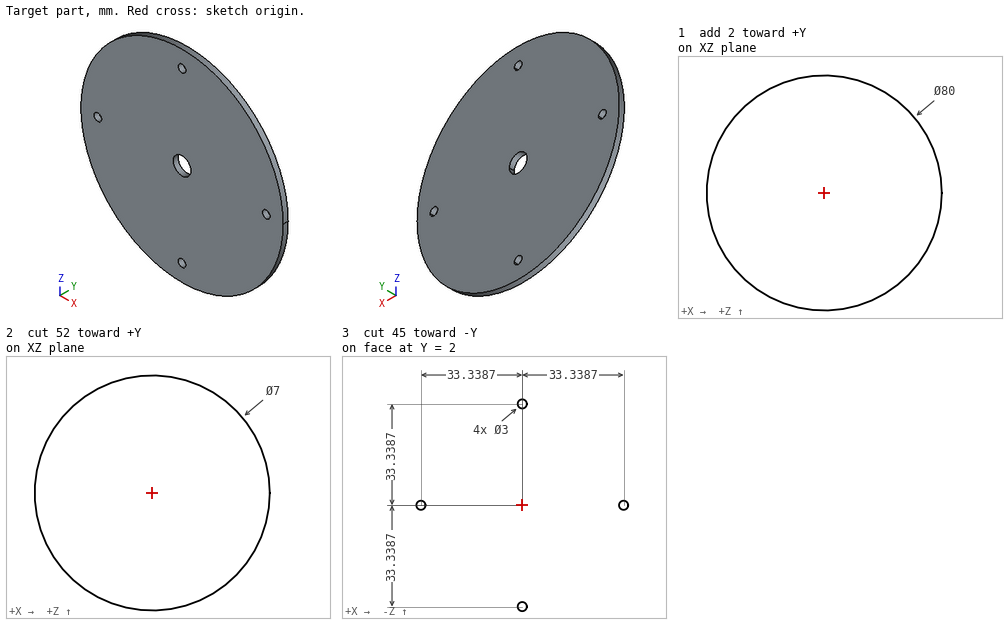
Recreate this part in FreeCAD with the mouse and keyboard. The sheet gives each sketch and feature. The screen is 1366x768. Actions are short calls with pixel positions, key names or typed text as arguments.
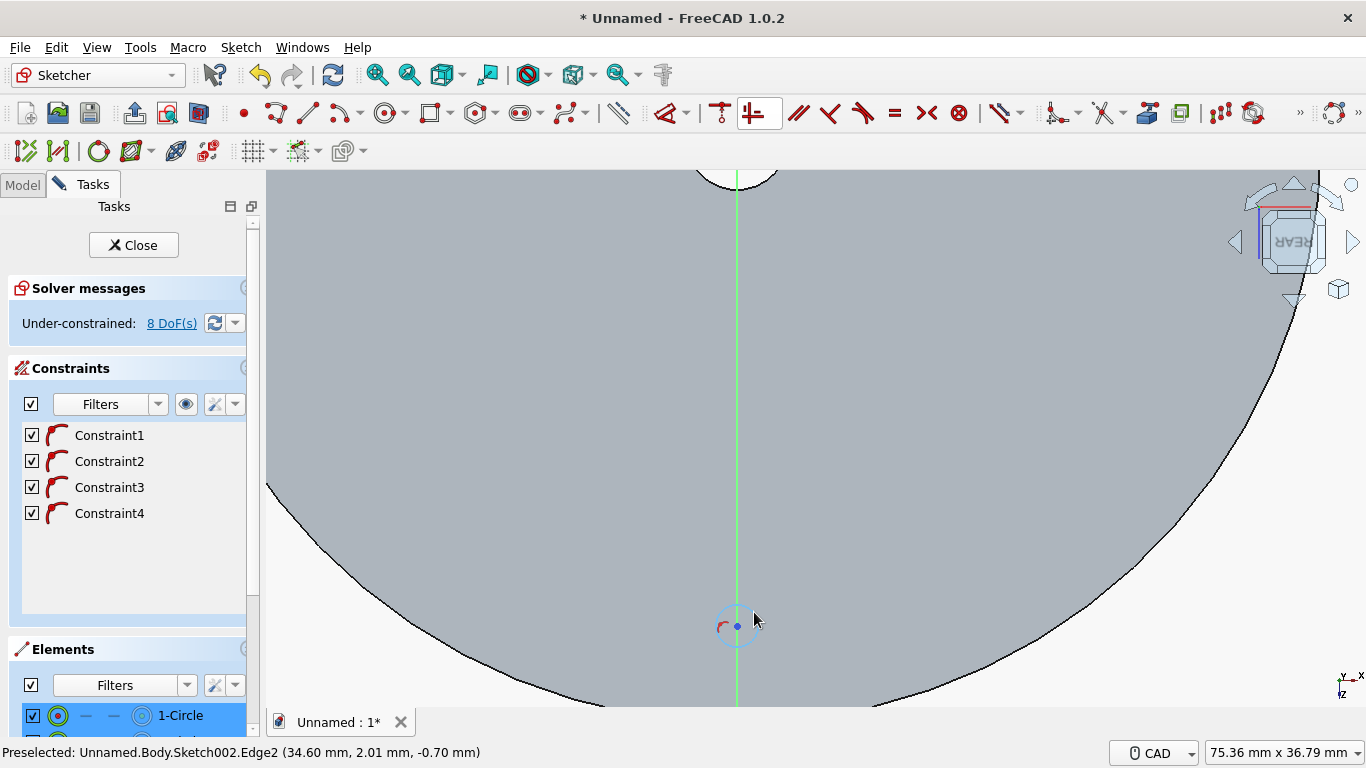
click(752, 611)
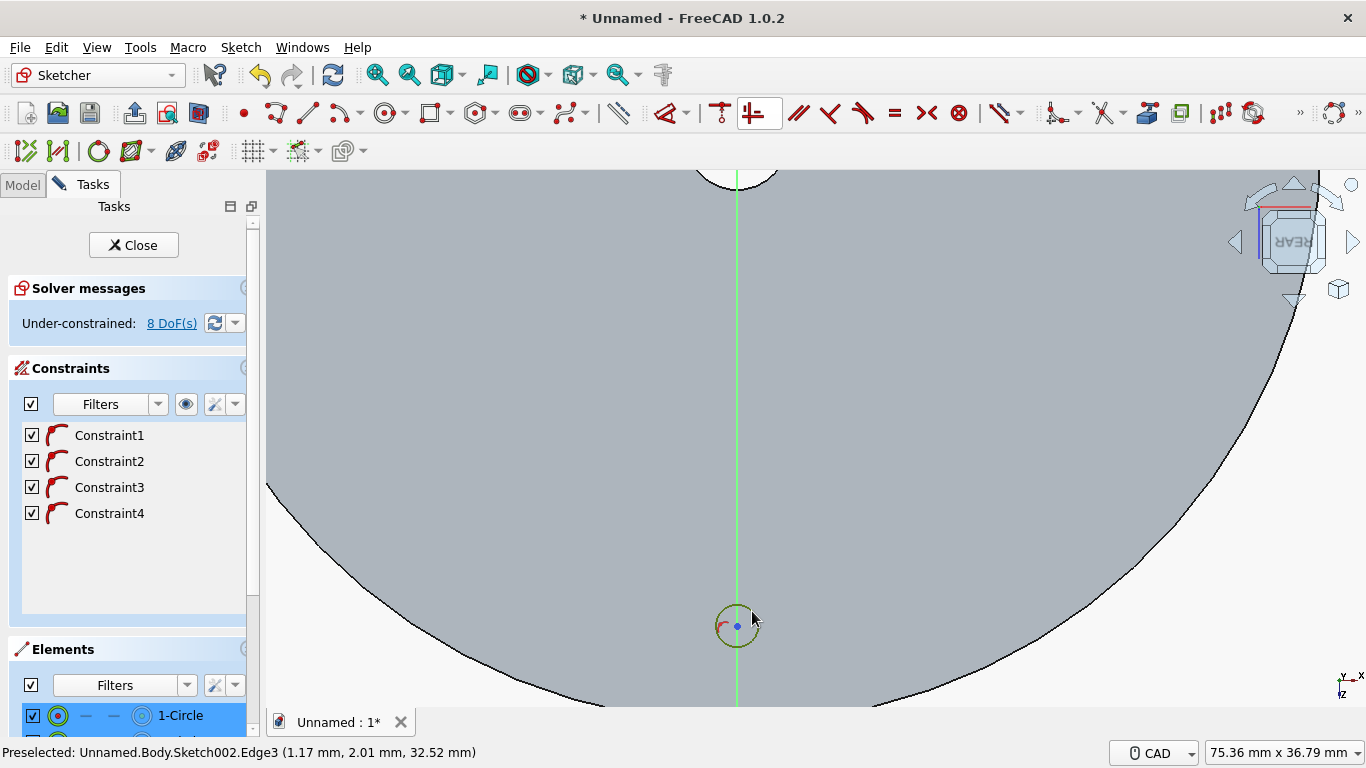
scroll(754, 613, down, 5)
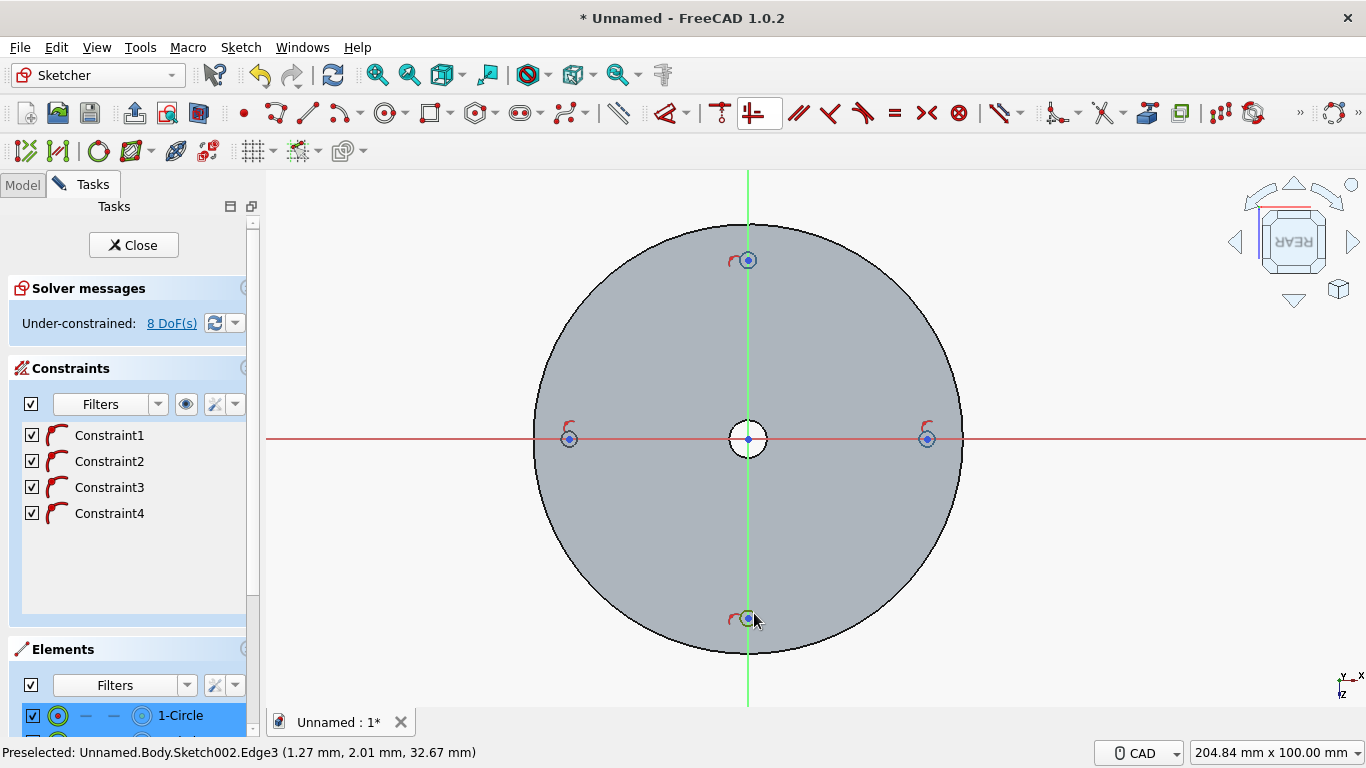
scroll(575, 434, up, 5)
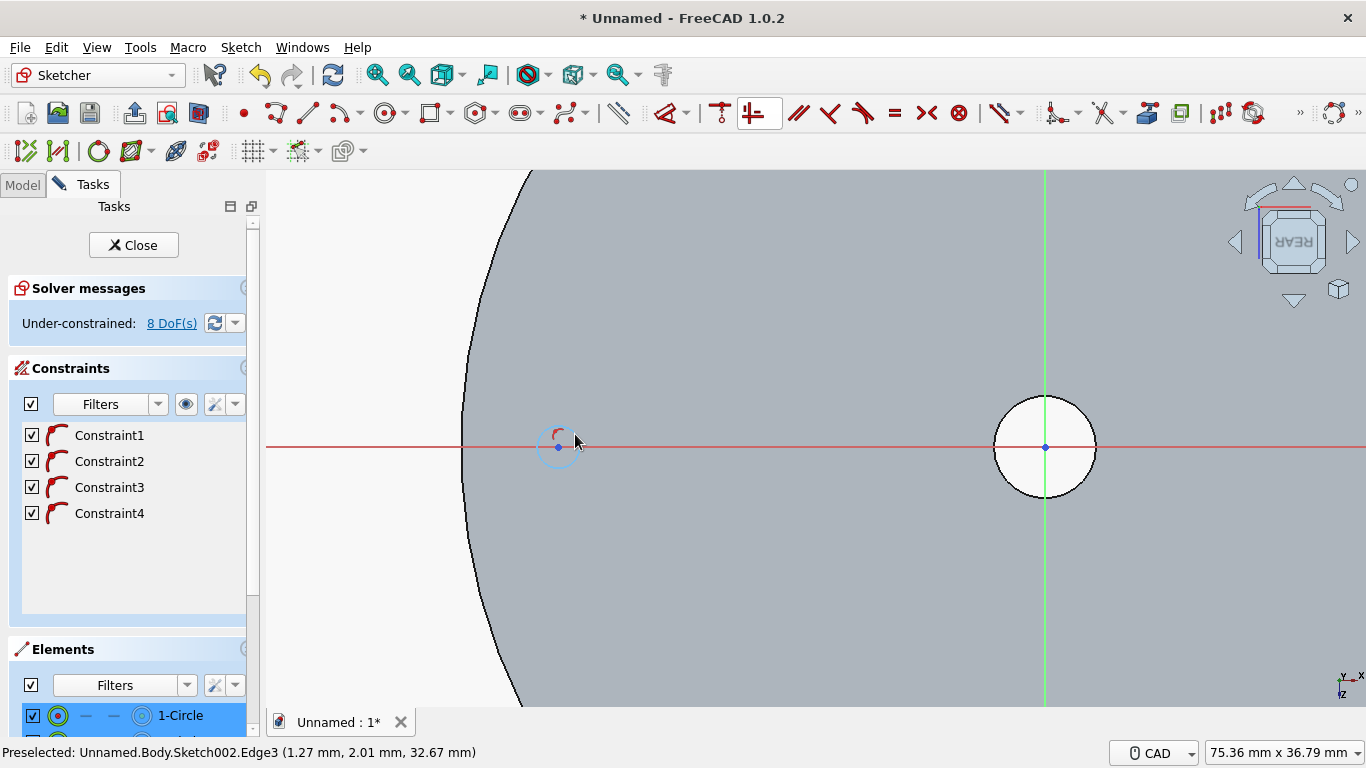
click(573, 432)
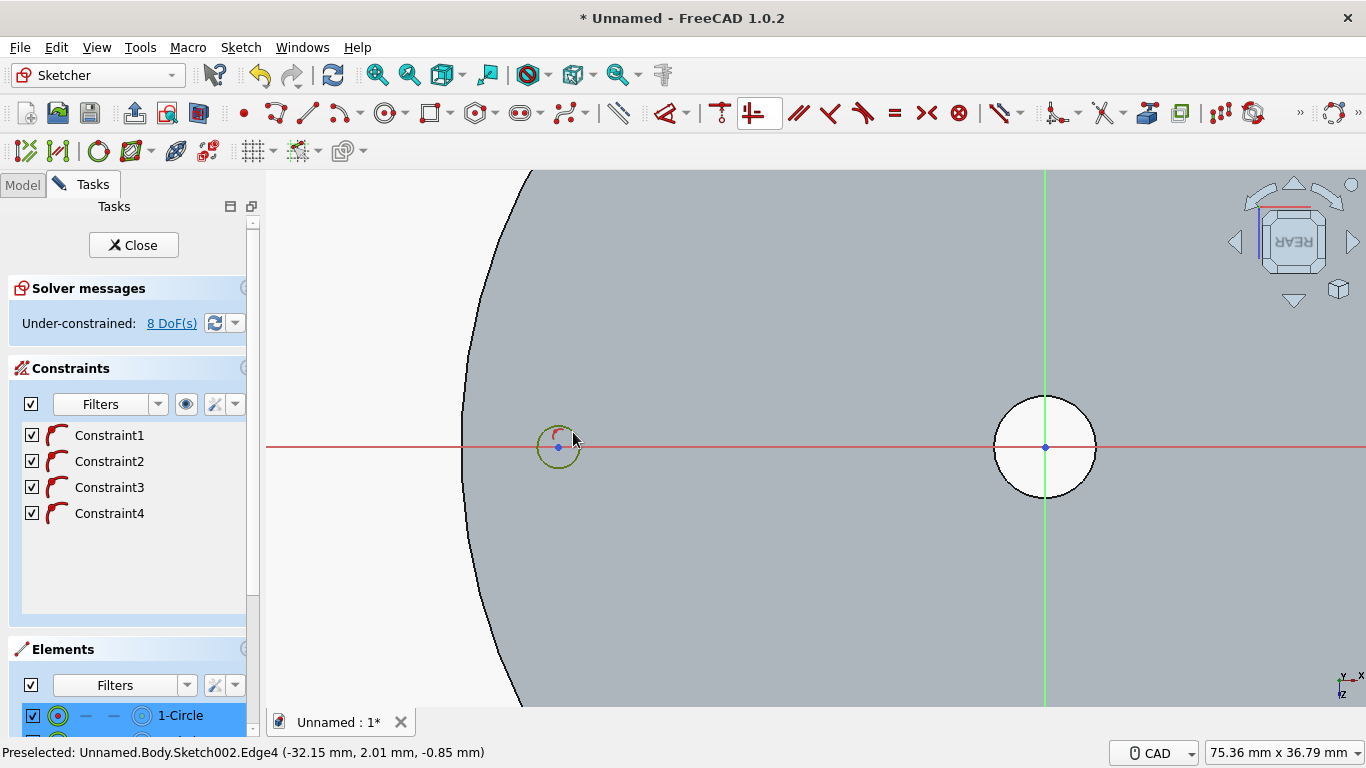
key(e)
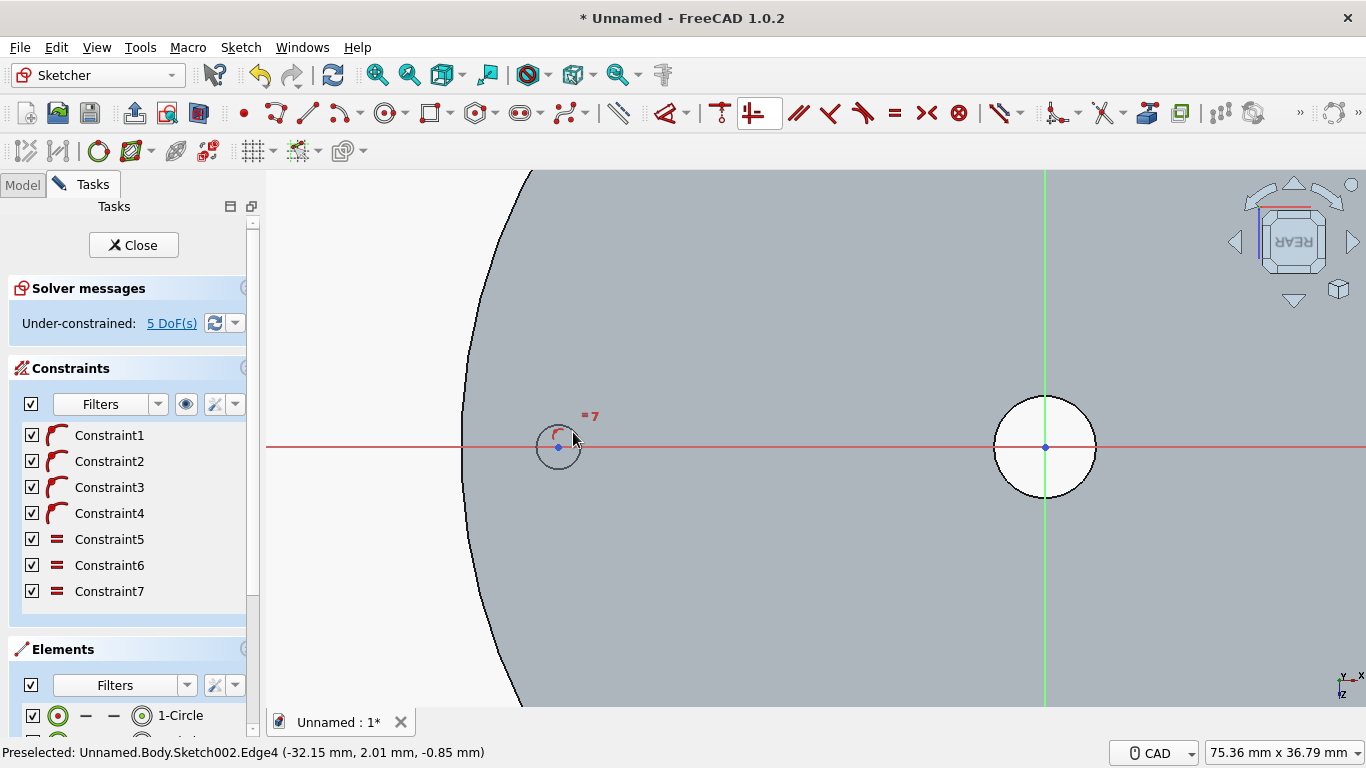
key(d)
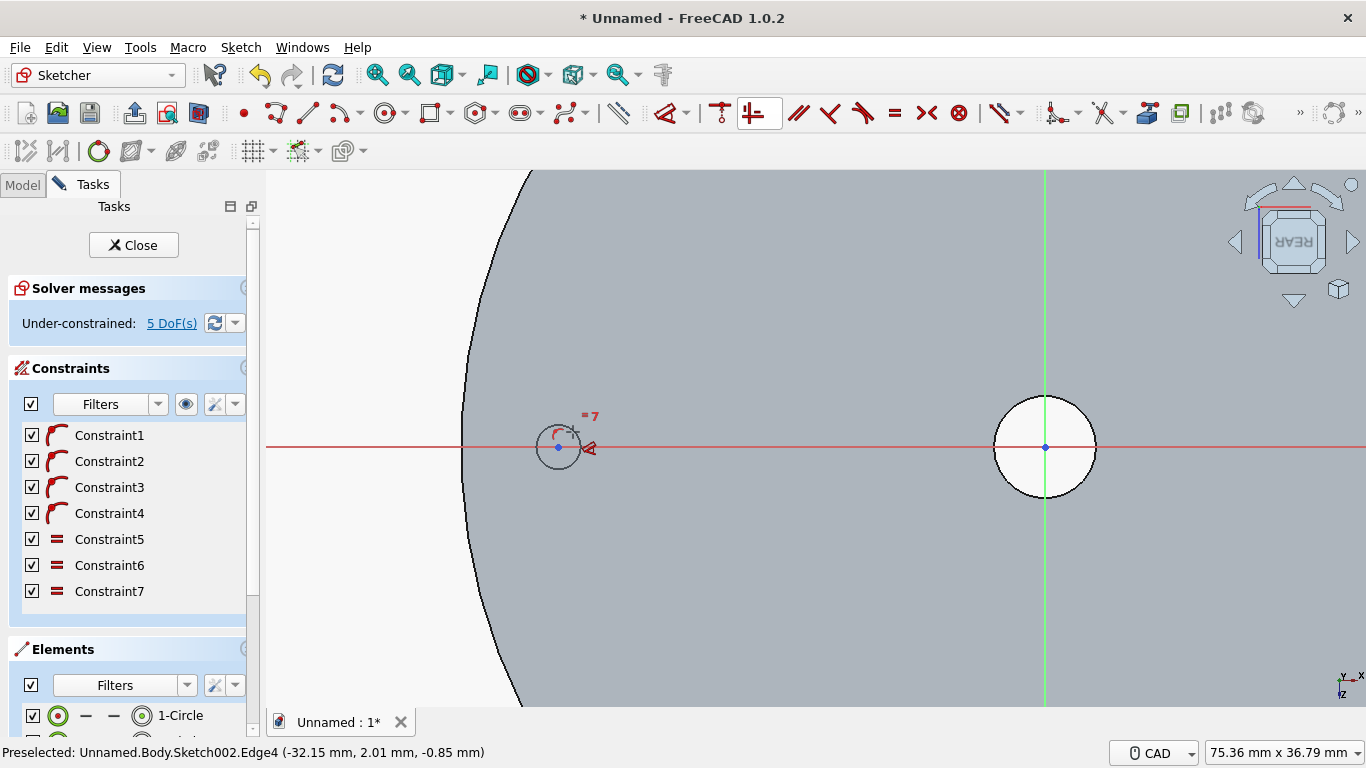
scroll(574, 433, down, 5)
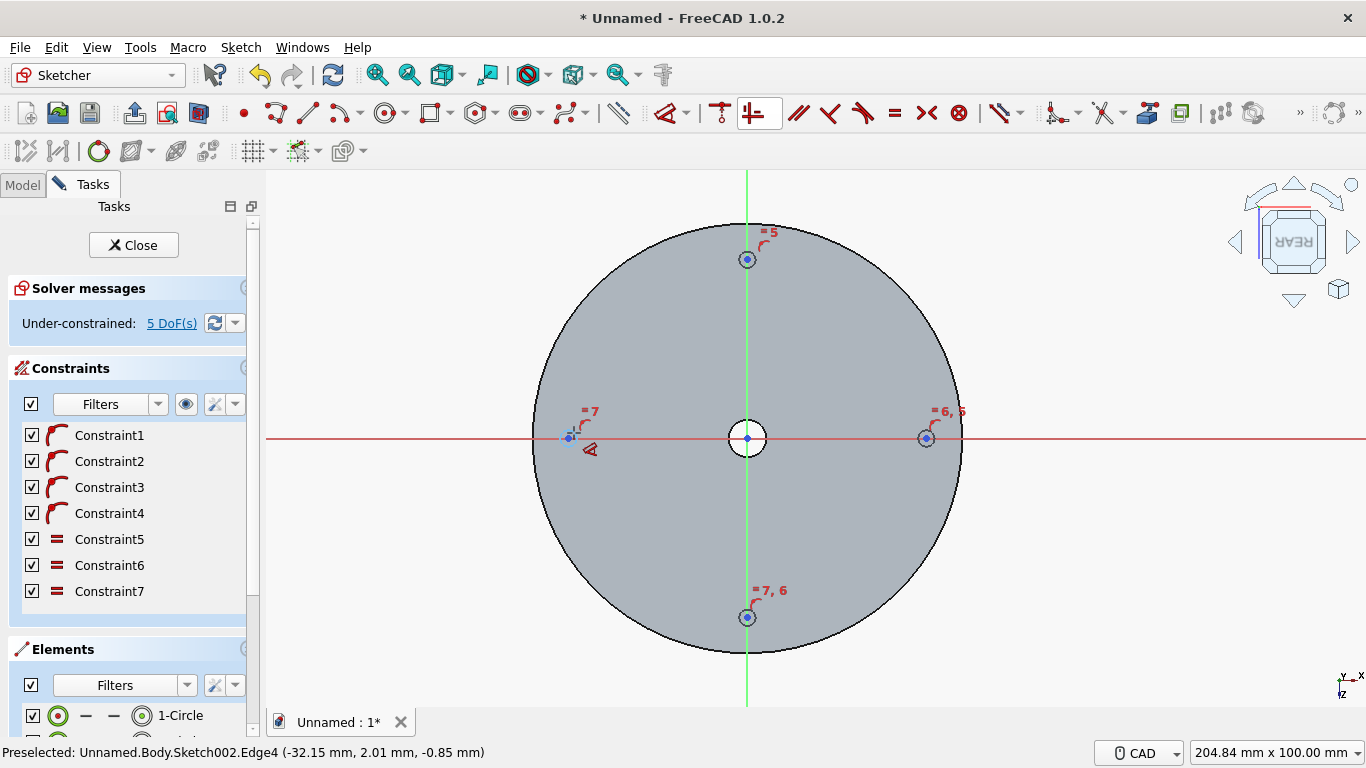
scroll(753, 254, up, 5)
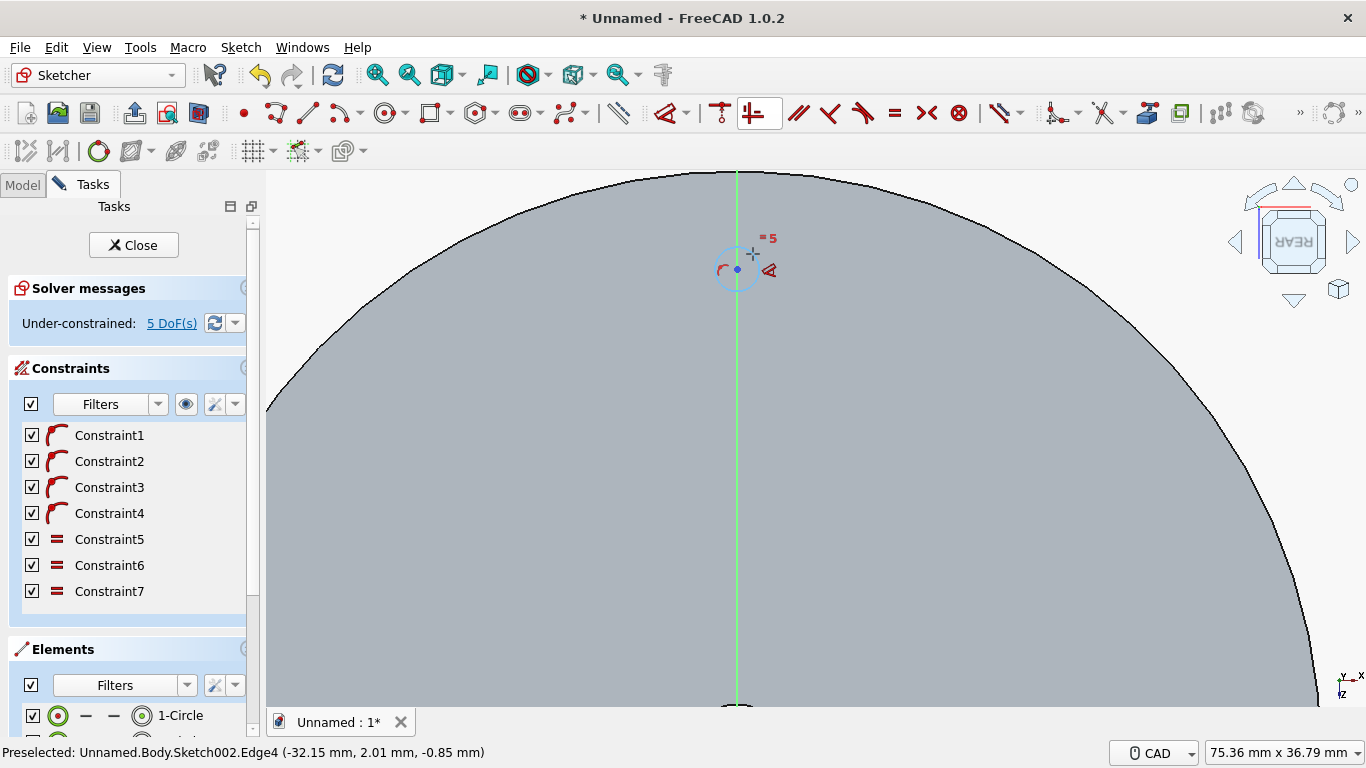
click(753, 254)
click(776, 232)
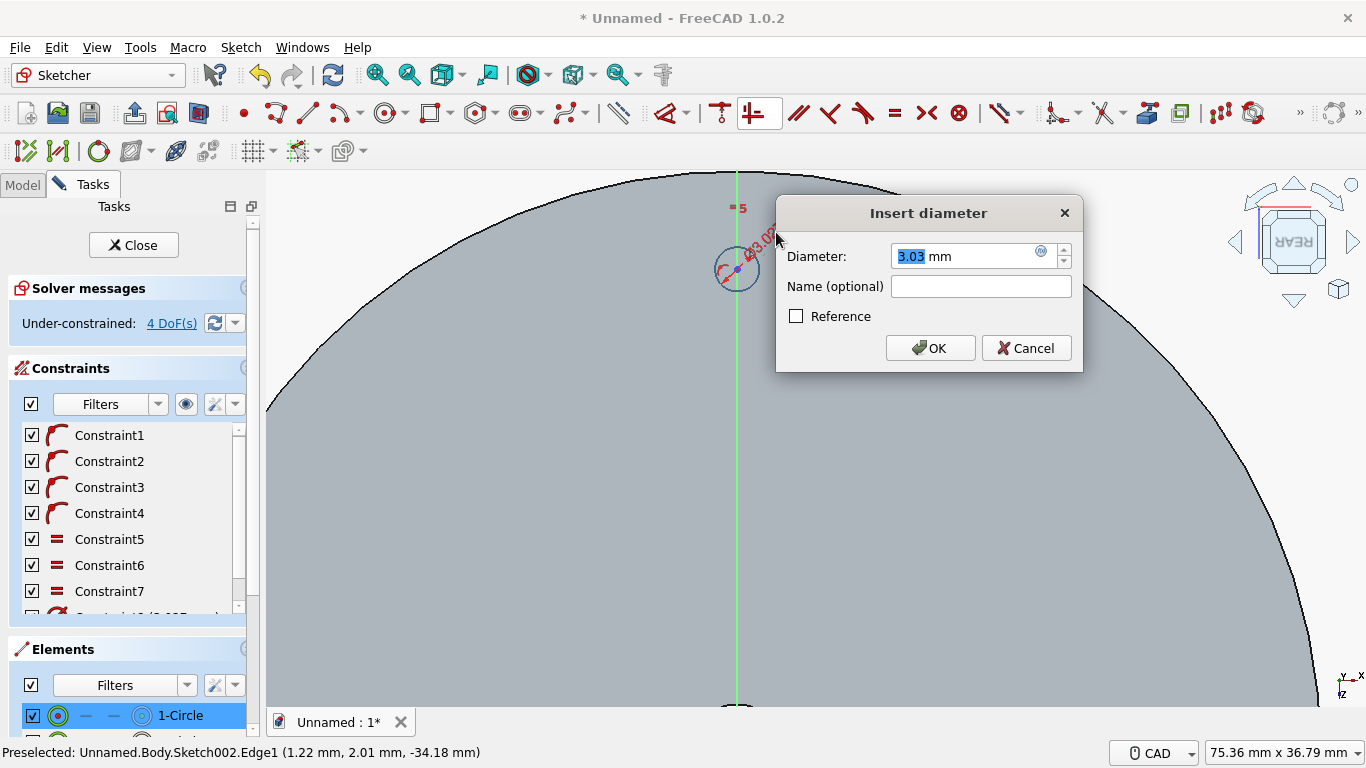
text(3)
key(Return)